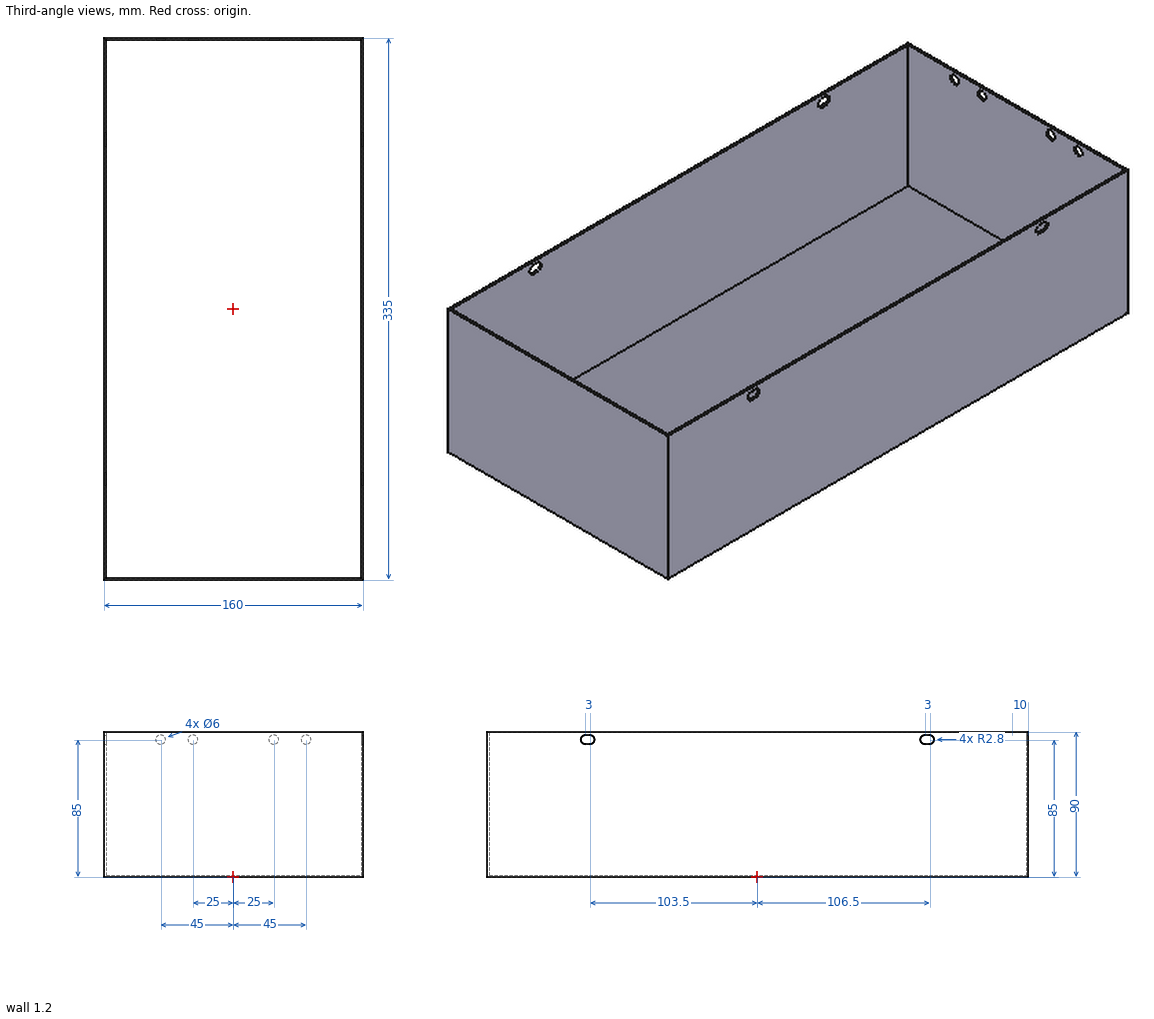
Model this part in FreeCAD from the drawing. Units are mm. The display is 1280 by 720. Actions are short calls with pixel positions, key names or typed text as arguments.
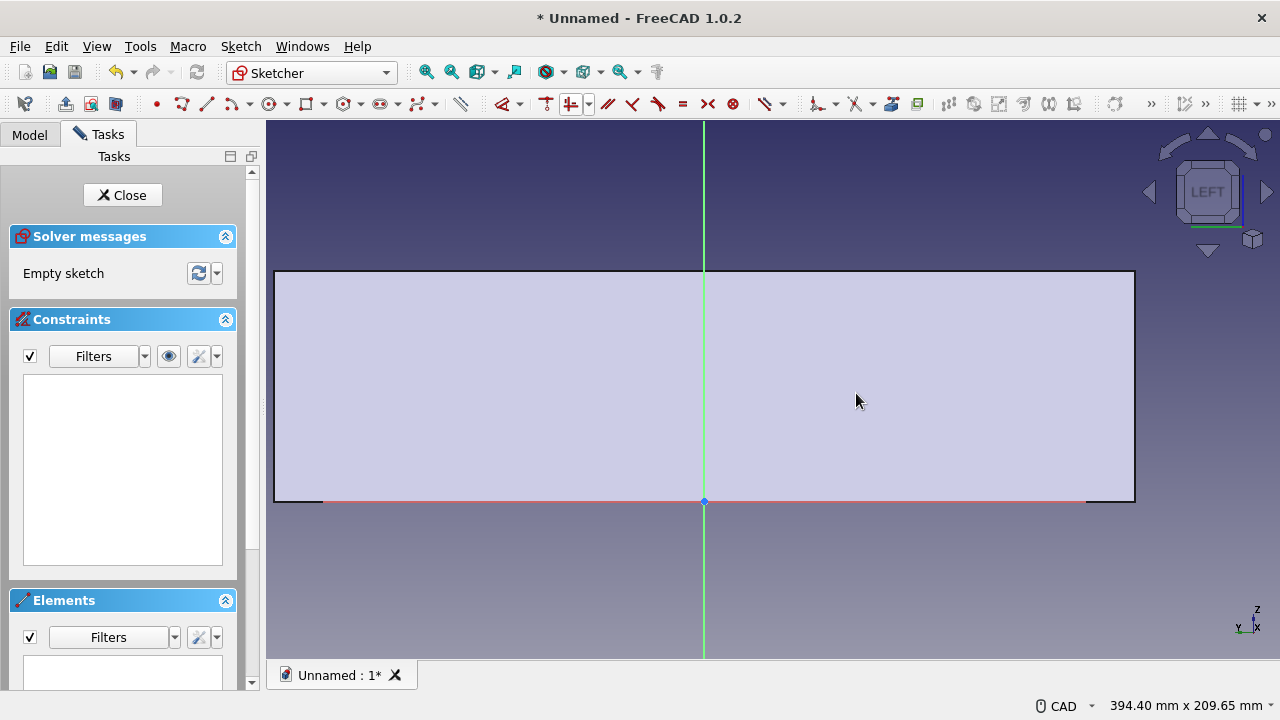
key(g)
key(s)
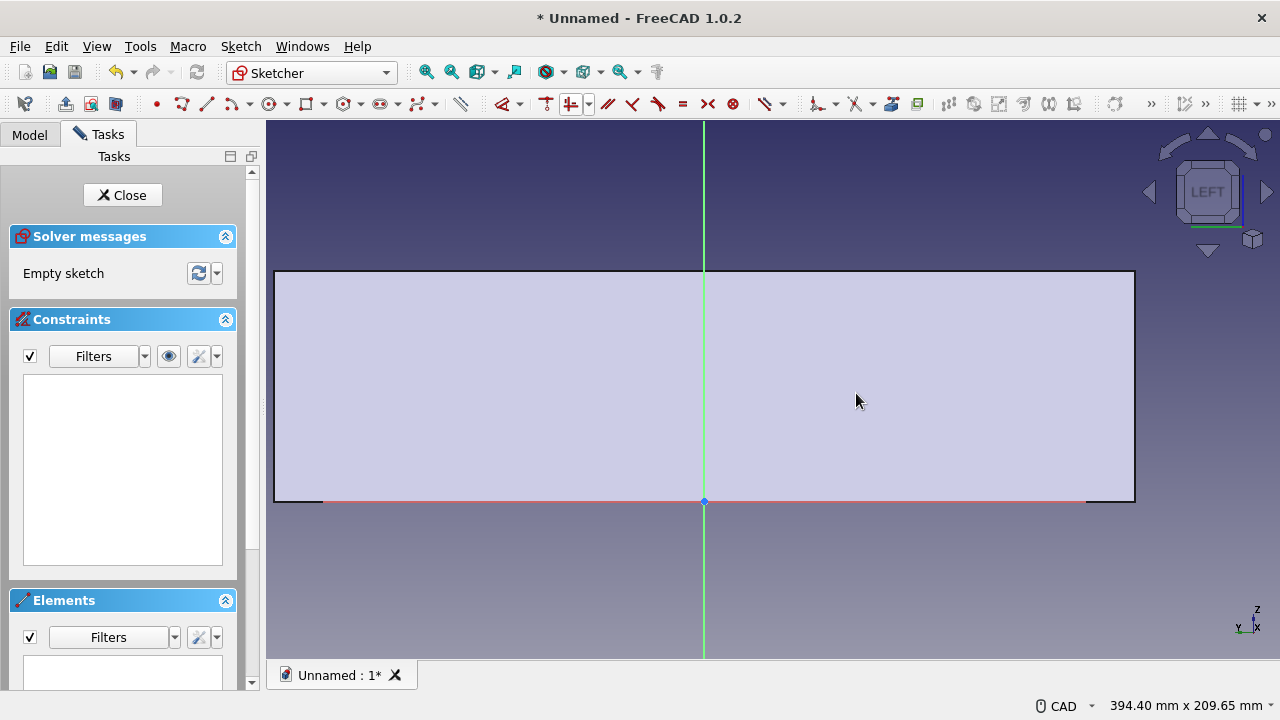
scroll(430, 283, up, 6)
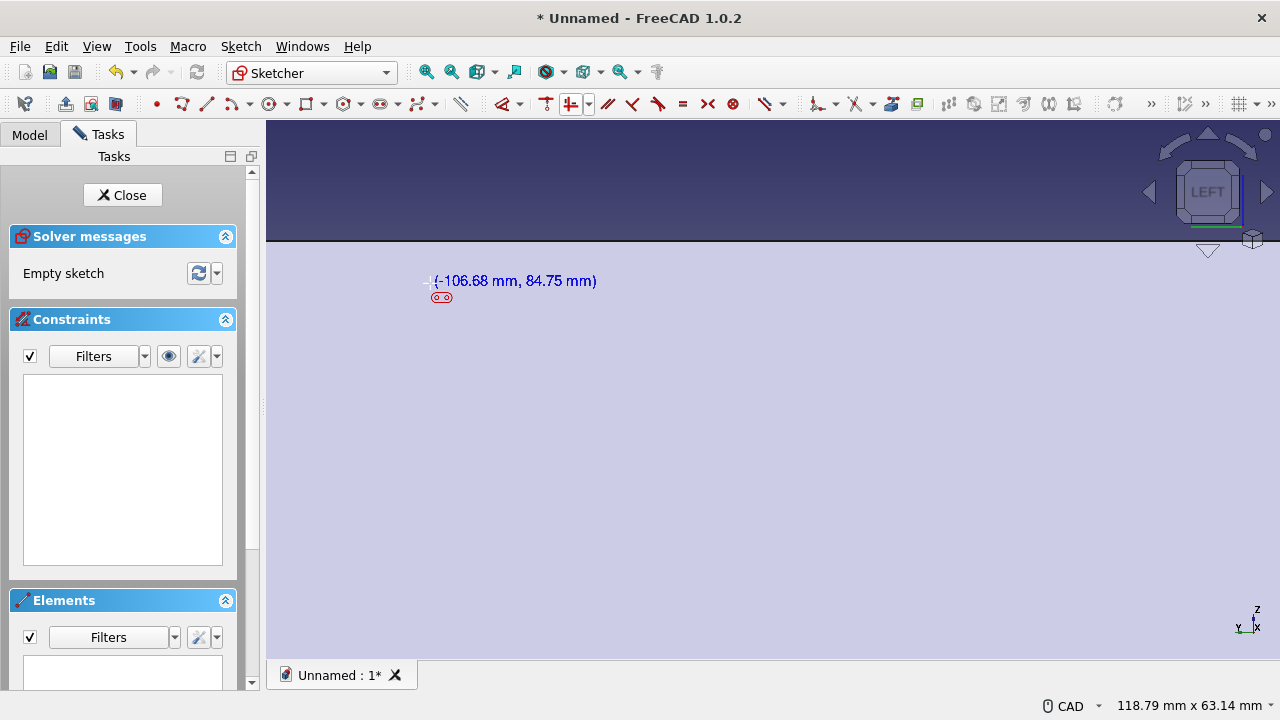
click(431, 284)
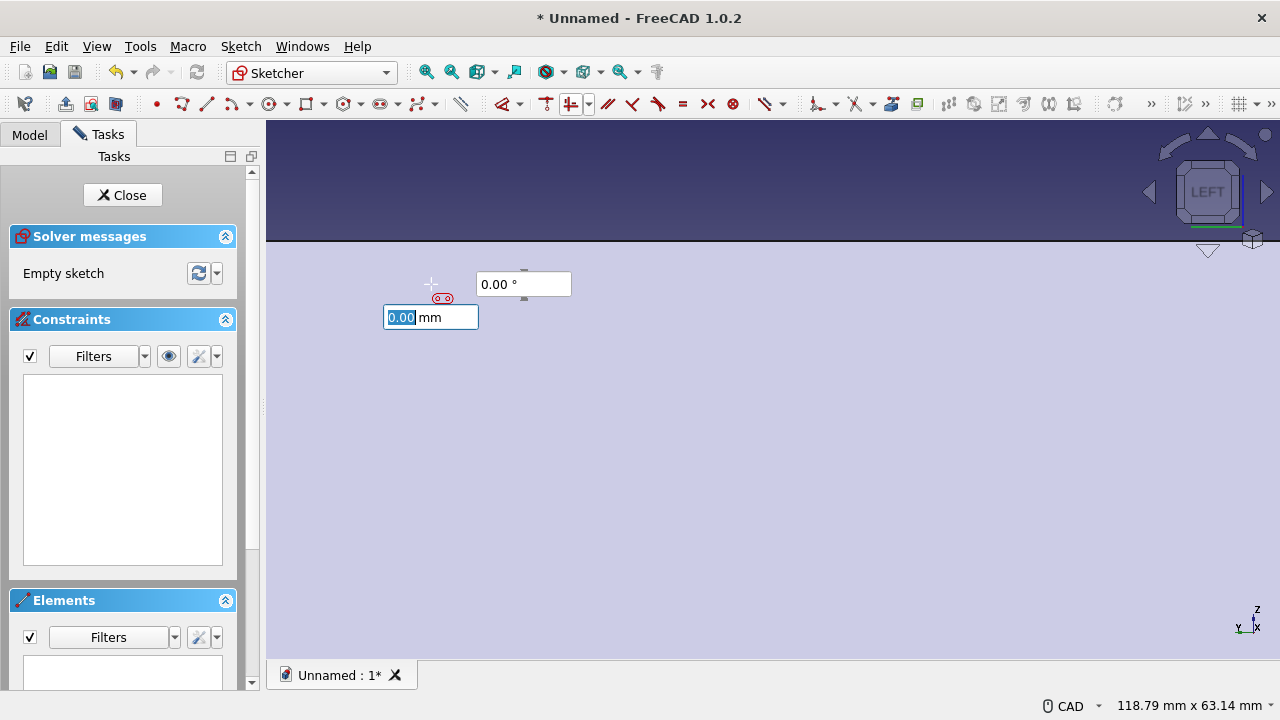
click(457, 284)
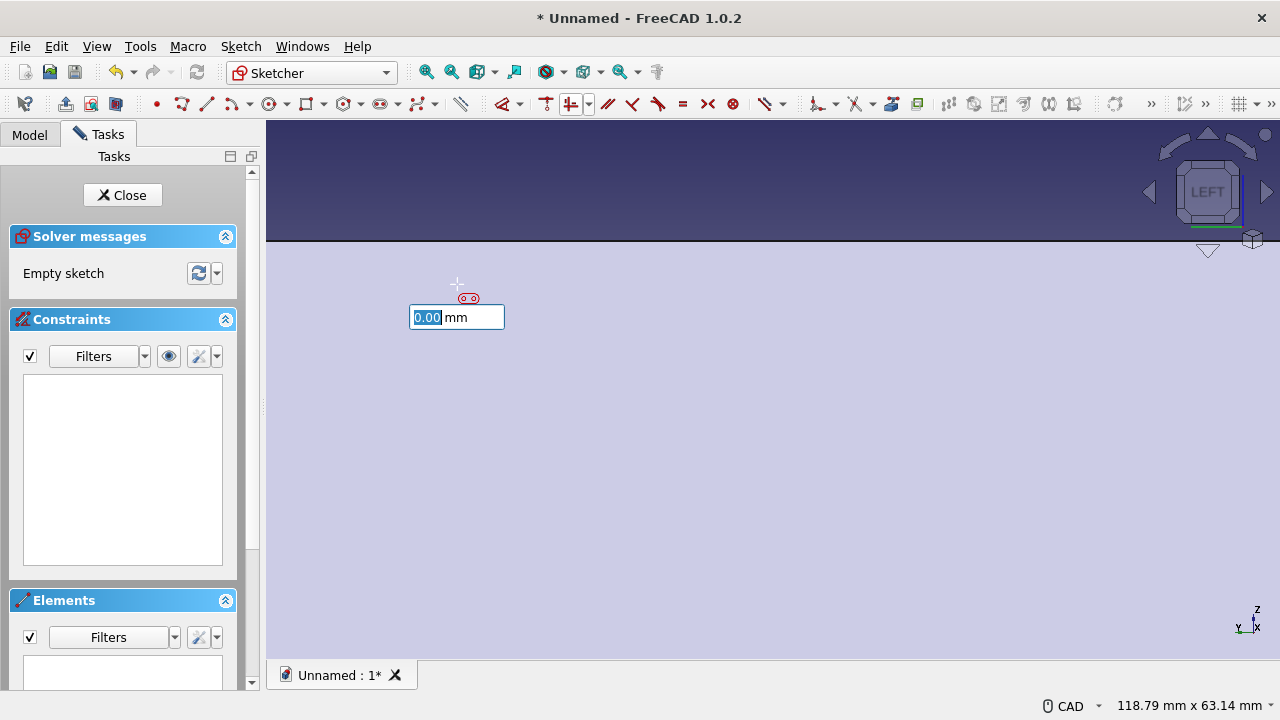
click(444, 260)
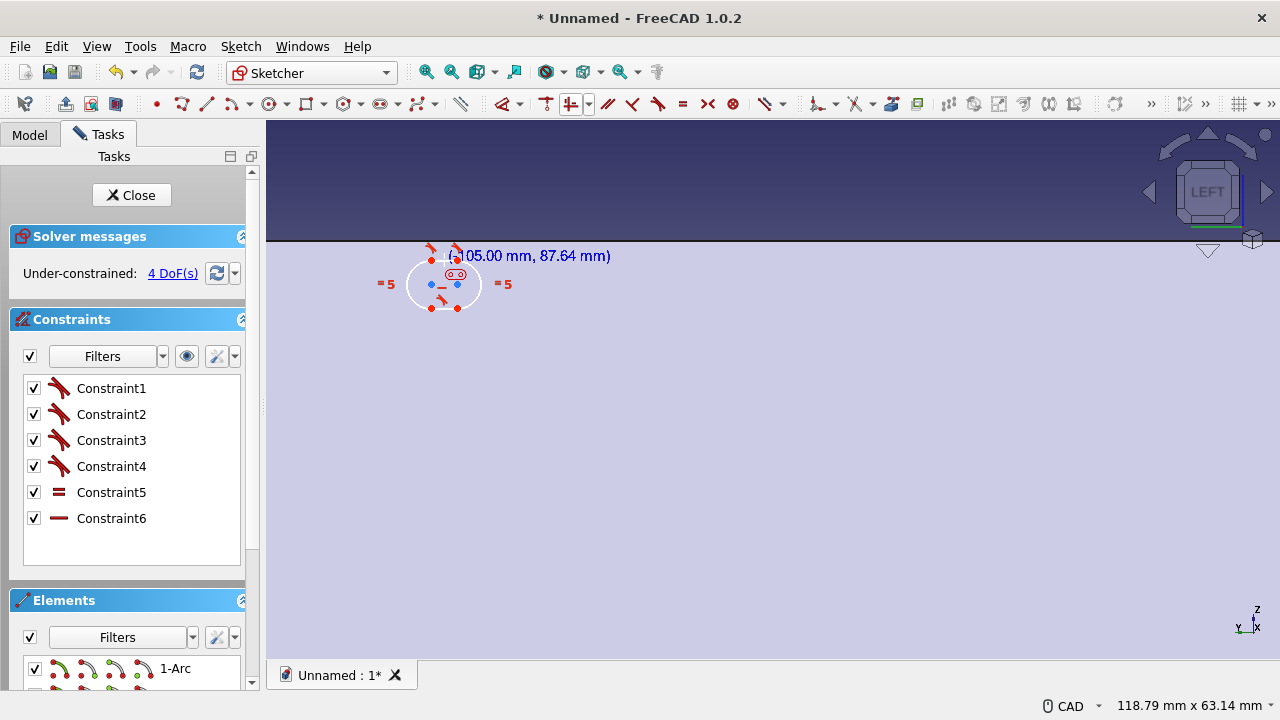
scroll(430, 284, down, 6)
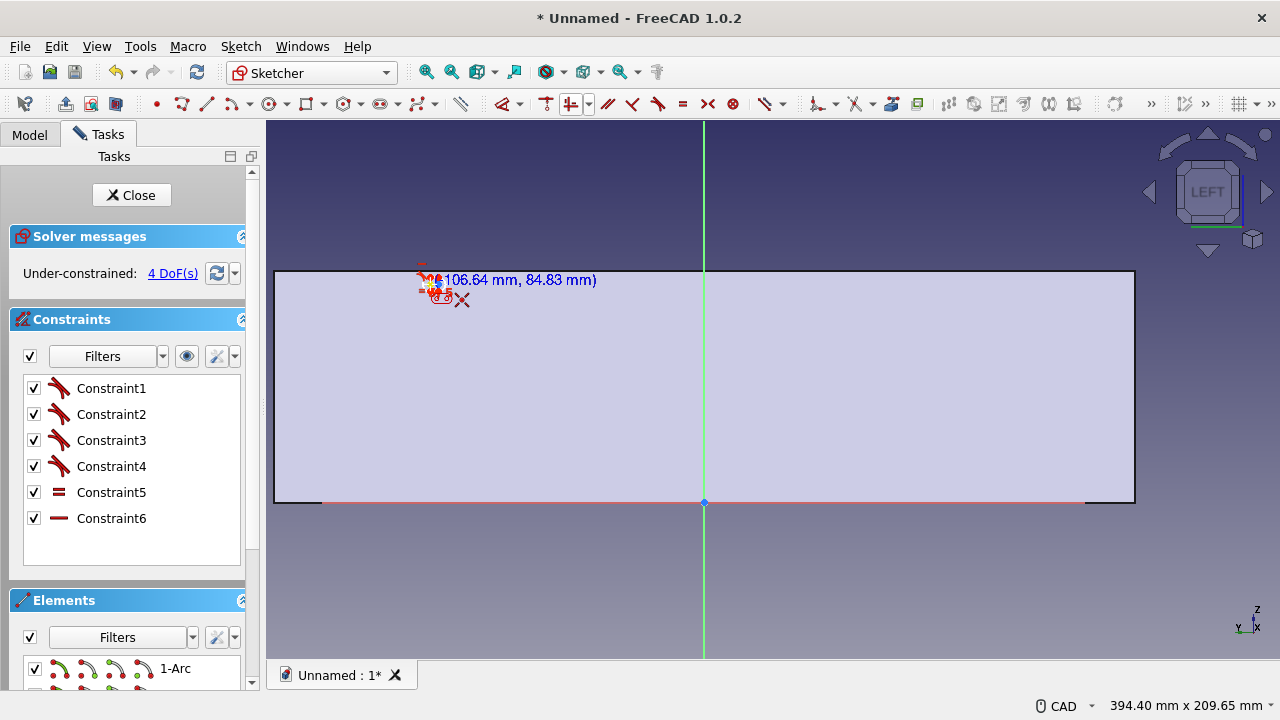
scroll(970, 284, up, 6)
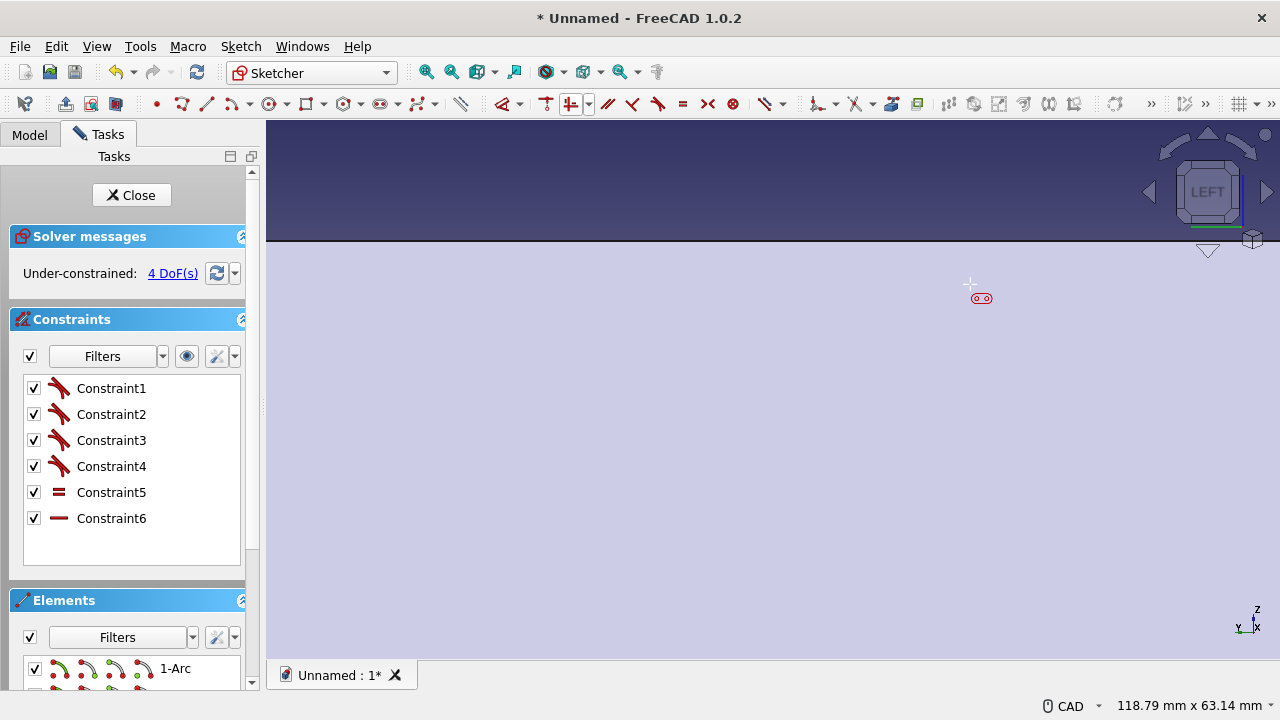
click(970, 284)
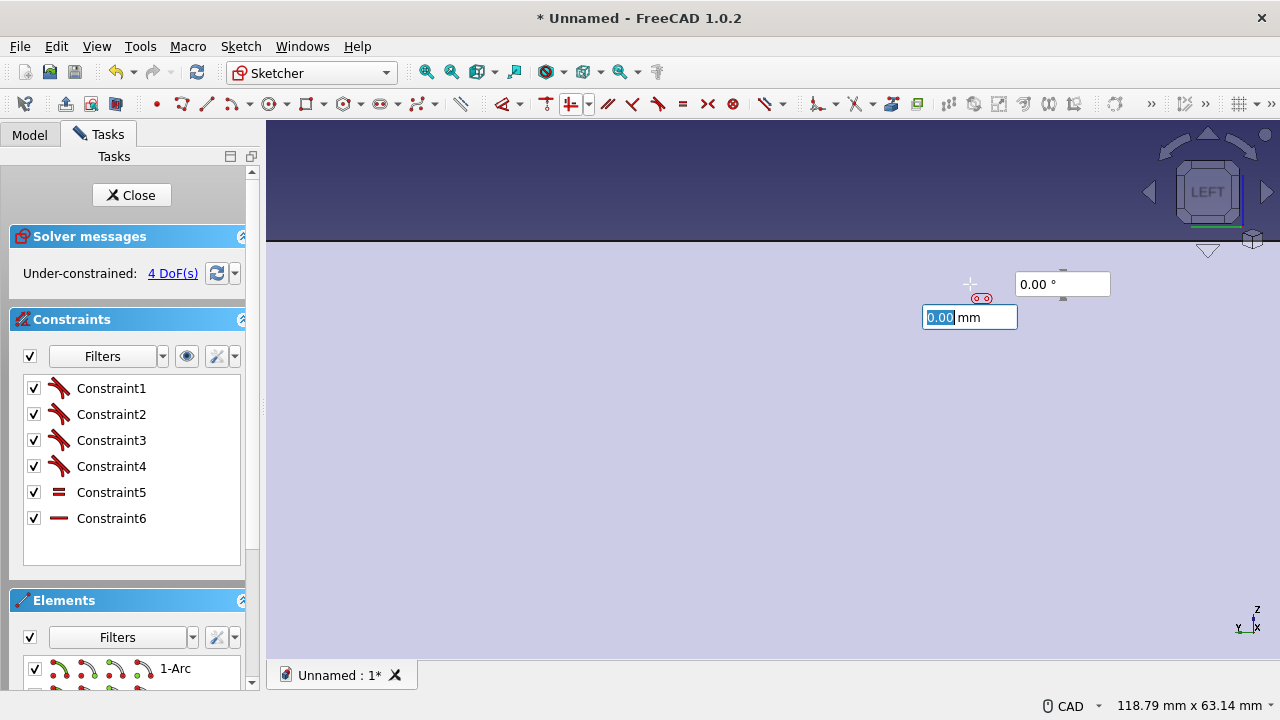
click(995, 284)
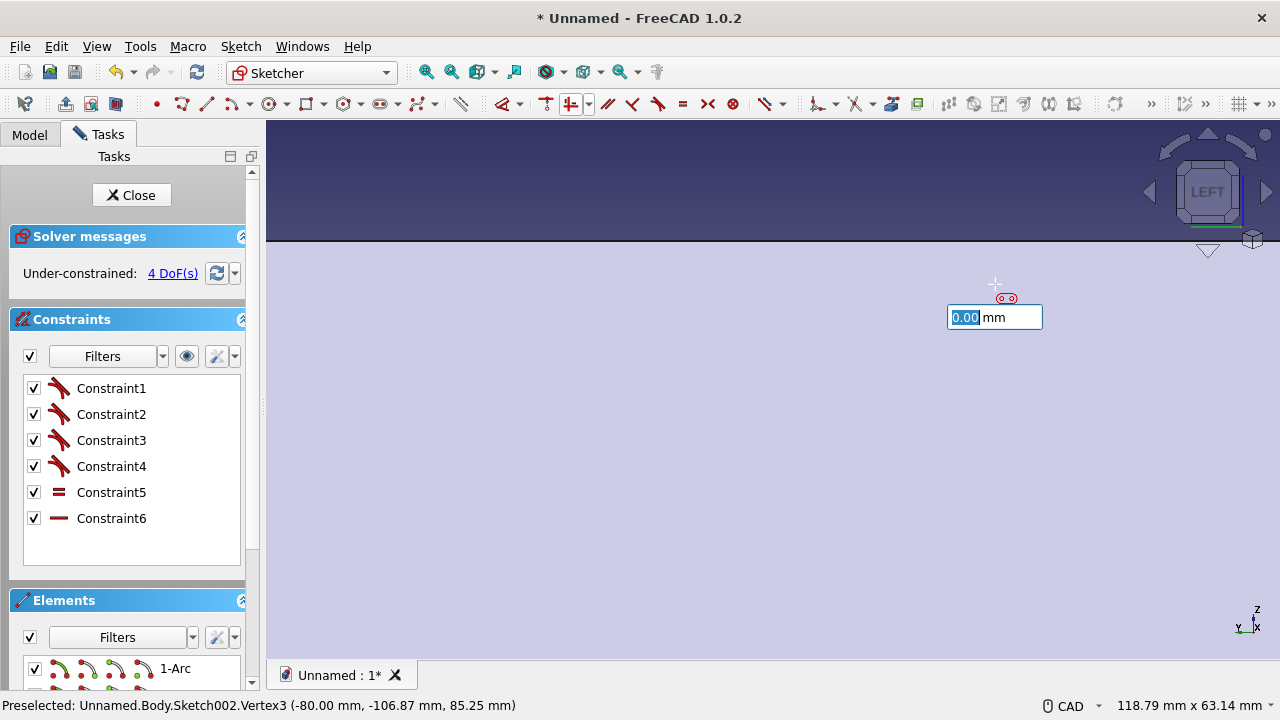
click(982, 260)
key(Escape)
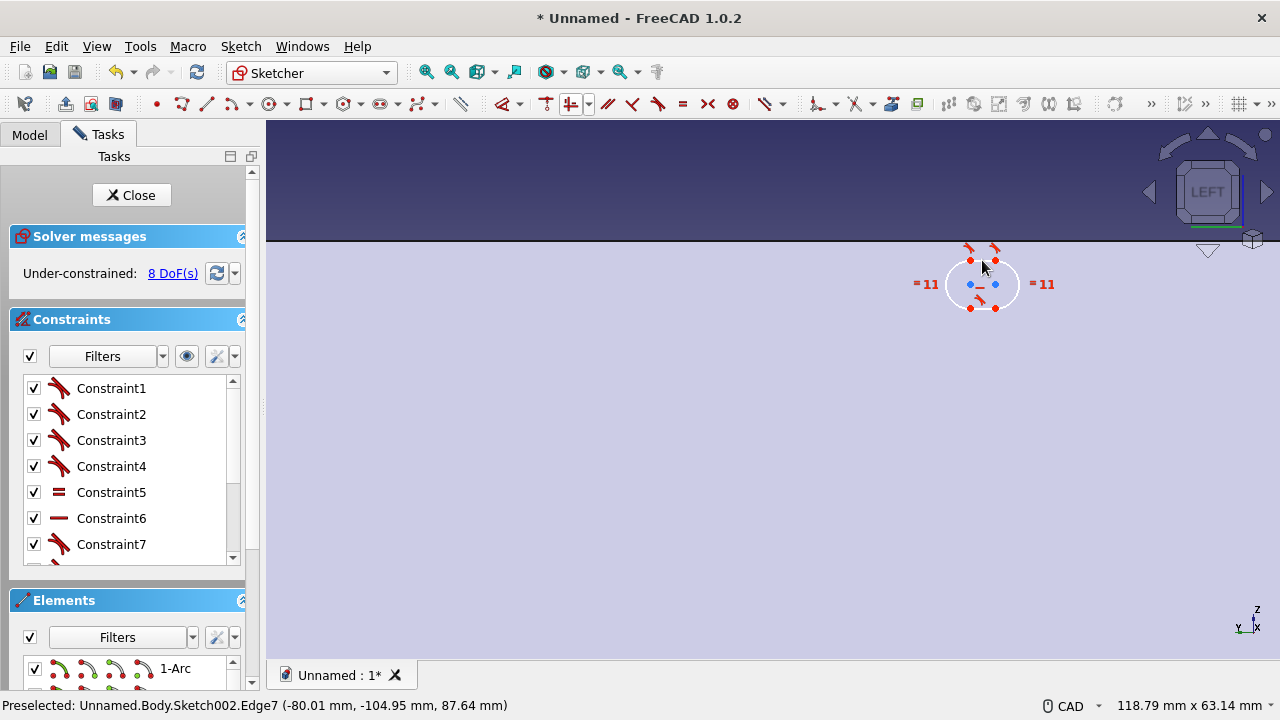
scroll(971, 284, down, 6)